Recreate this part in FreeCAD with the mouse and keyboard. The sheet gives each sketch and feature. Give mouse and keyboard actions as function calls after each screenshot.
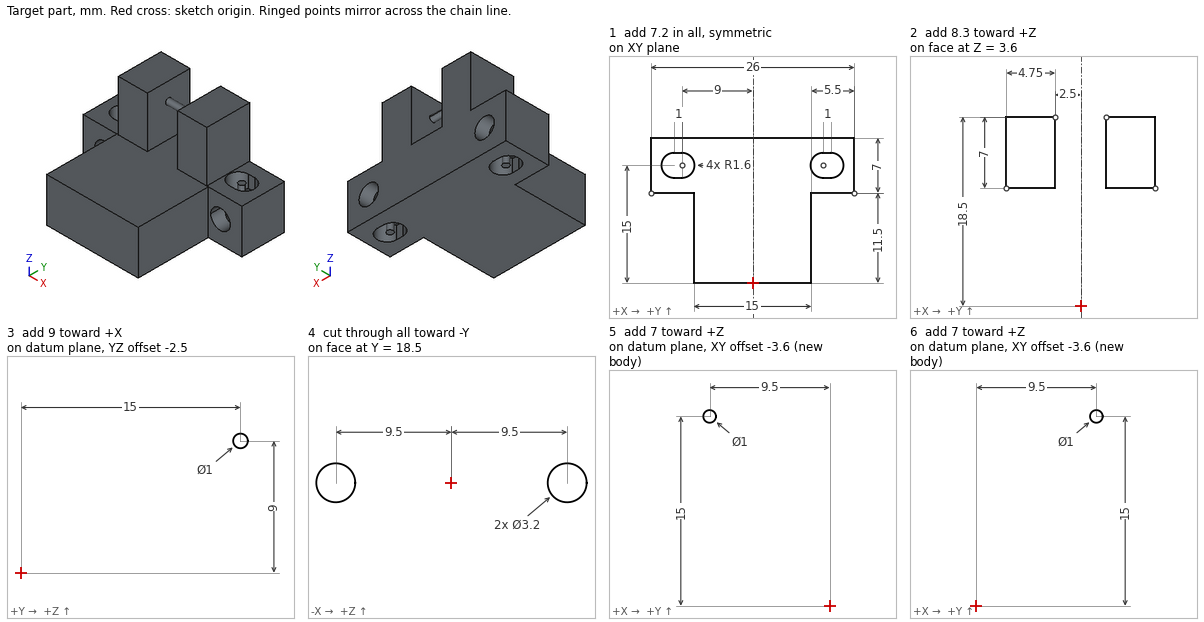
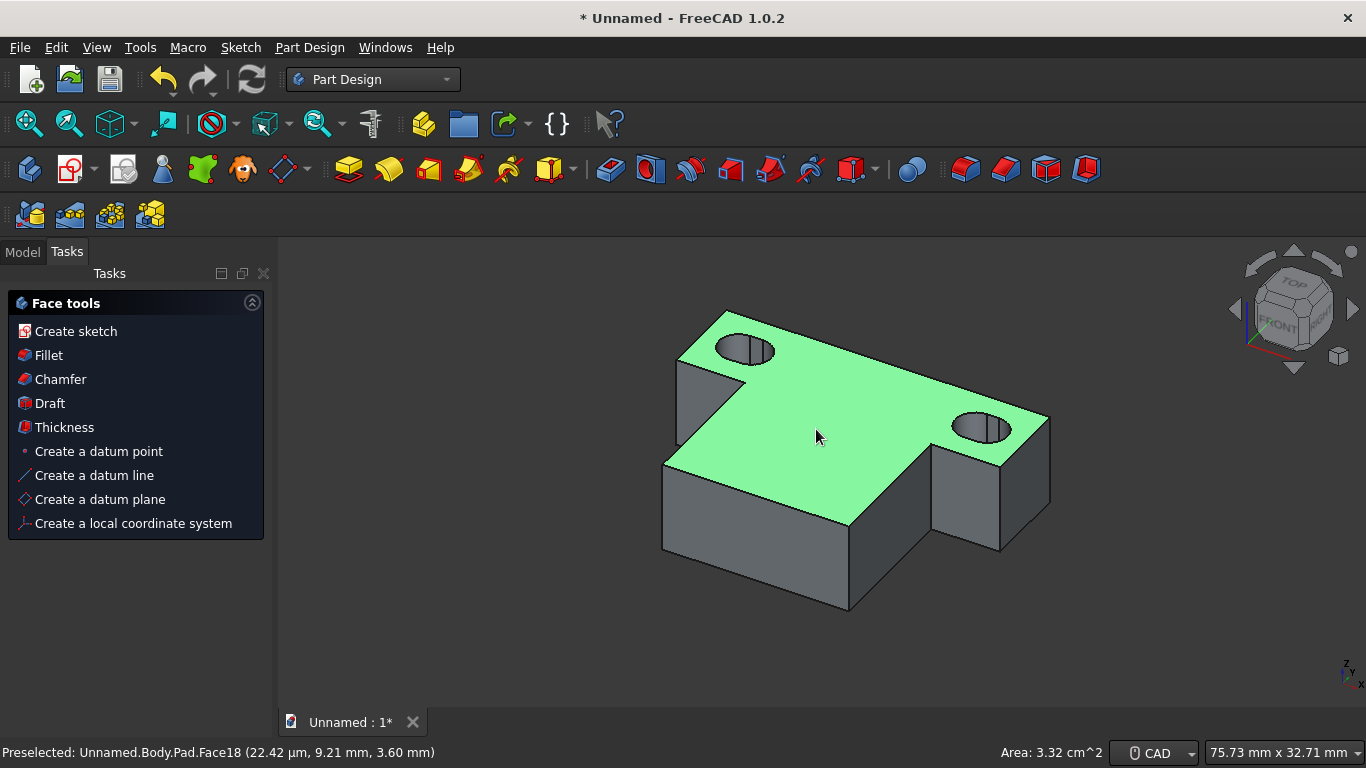
click(70, 170)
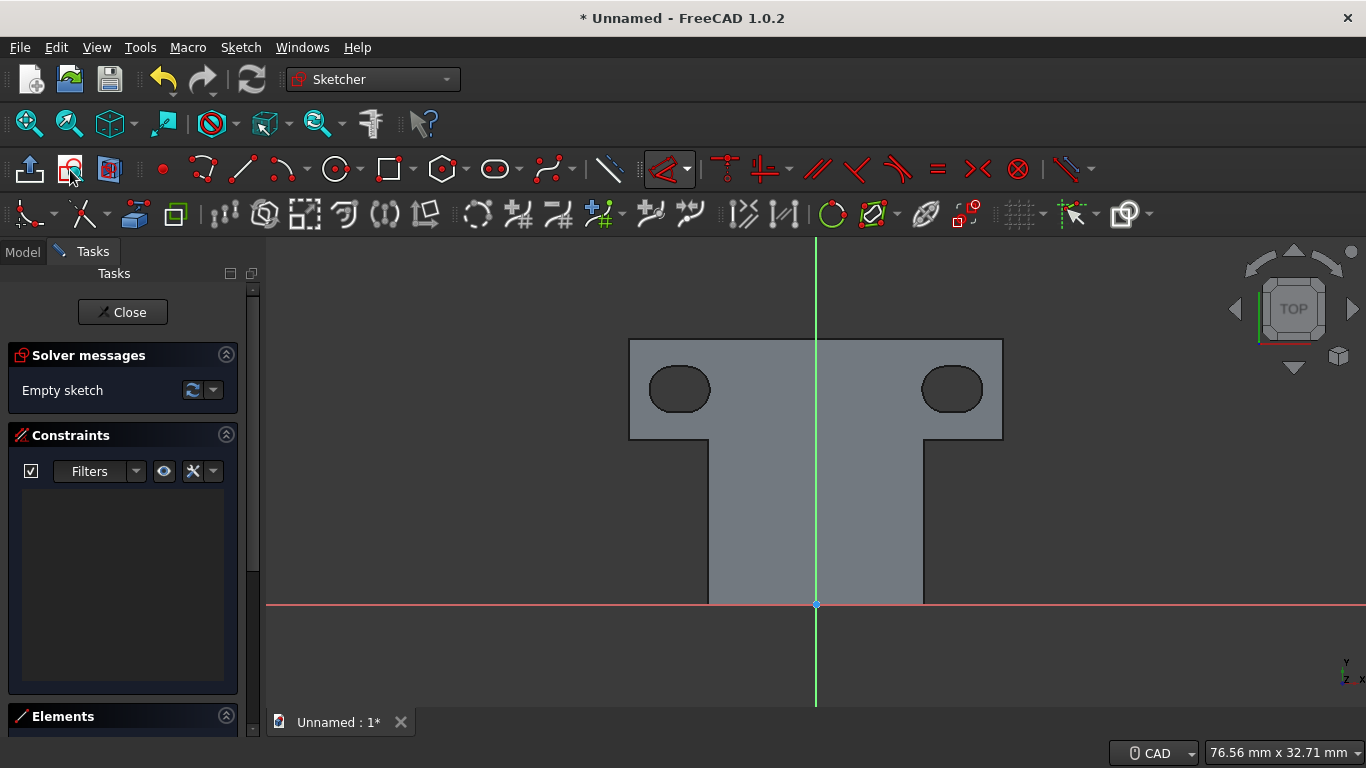
click(390, 170)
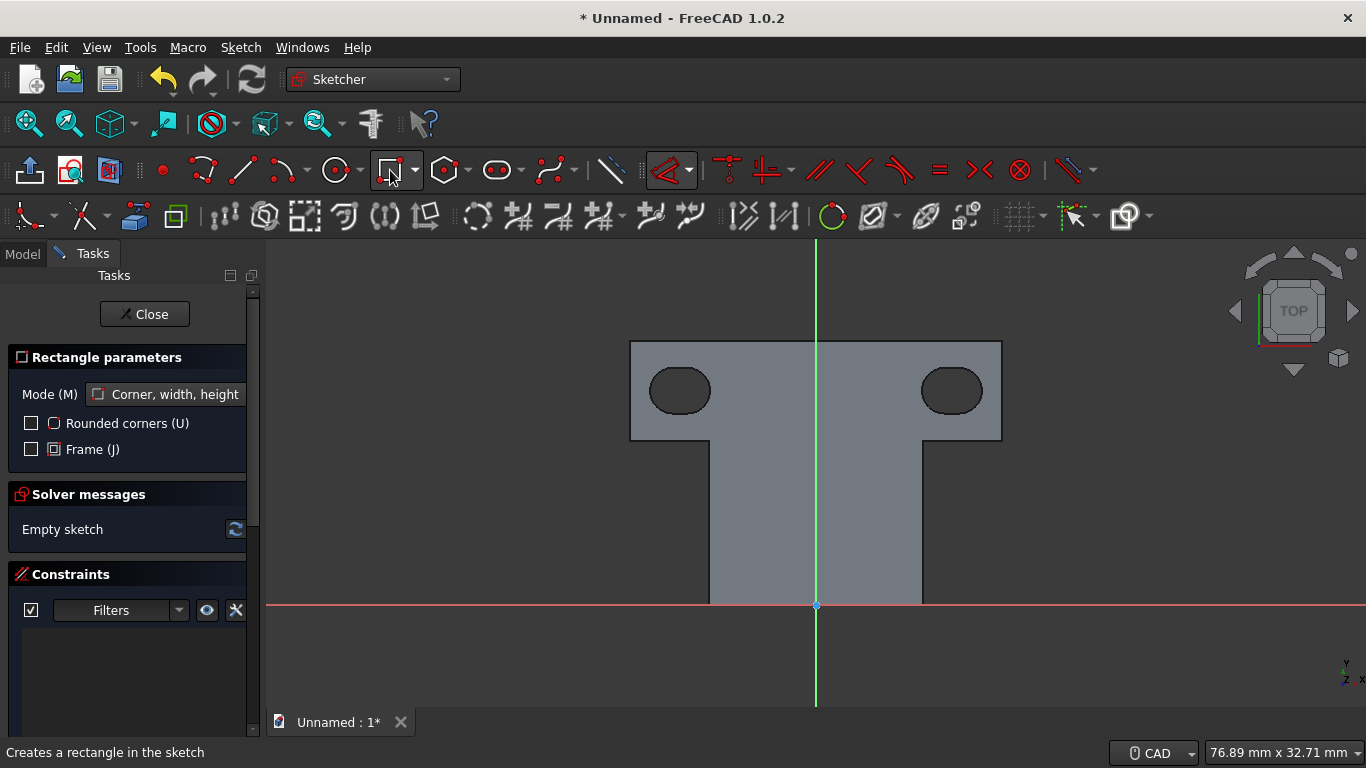
click(712, 341)
click(780, 441)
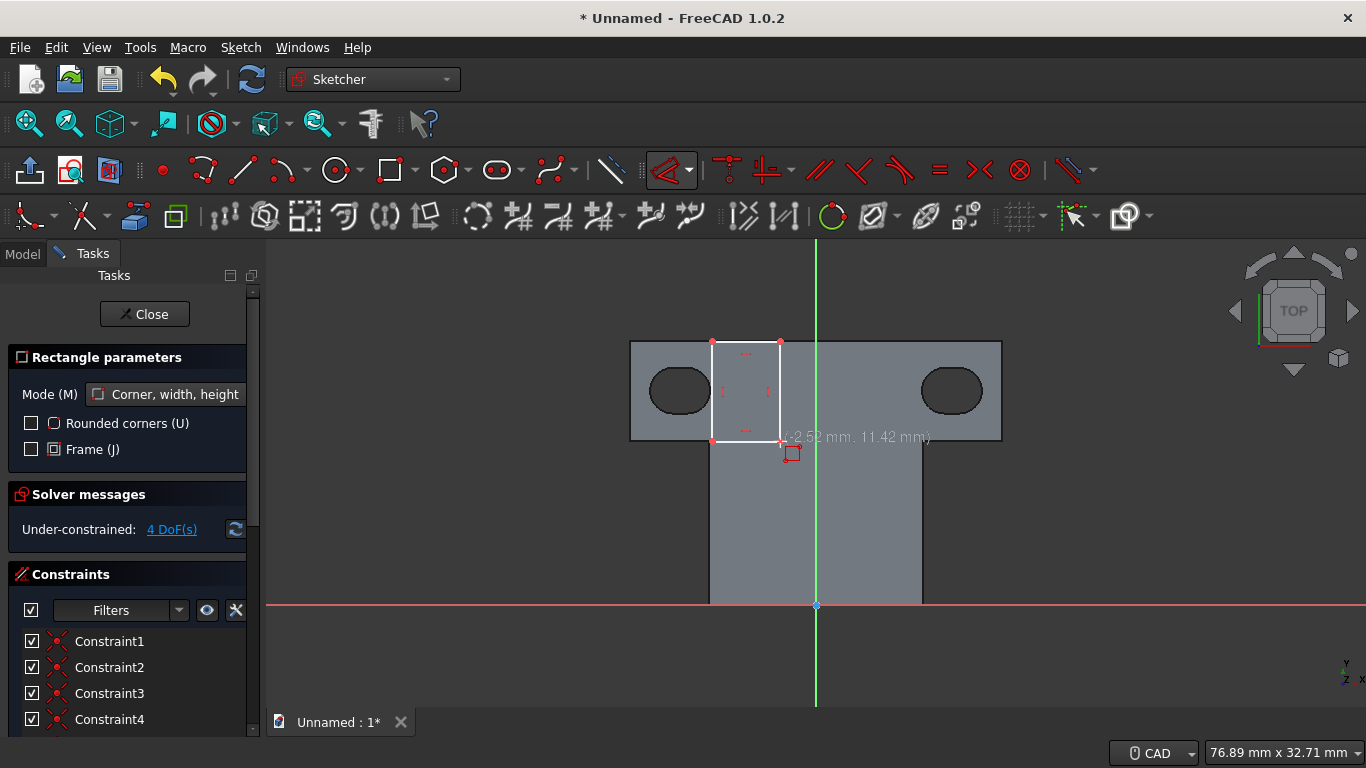
click(852, 341)
click(920, 441)
key(Escape)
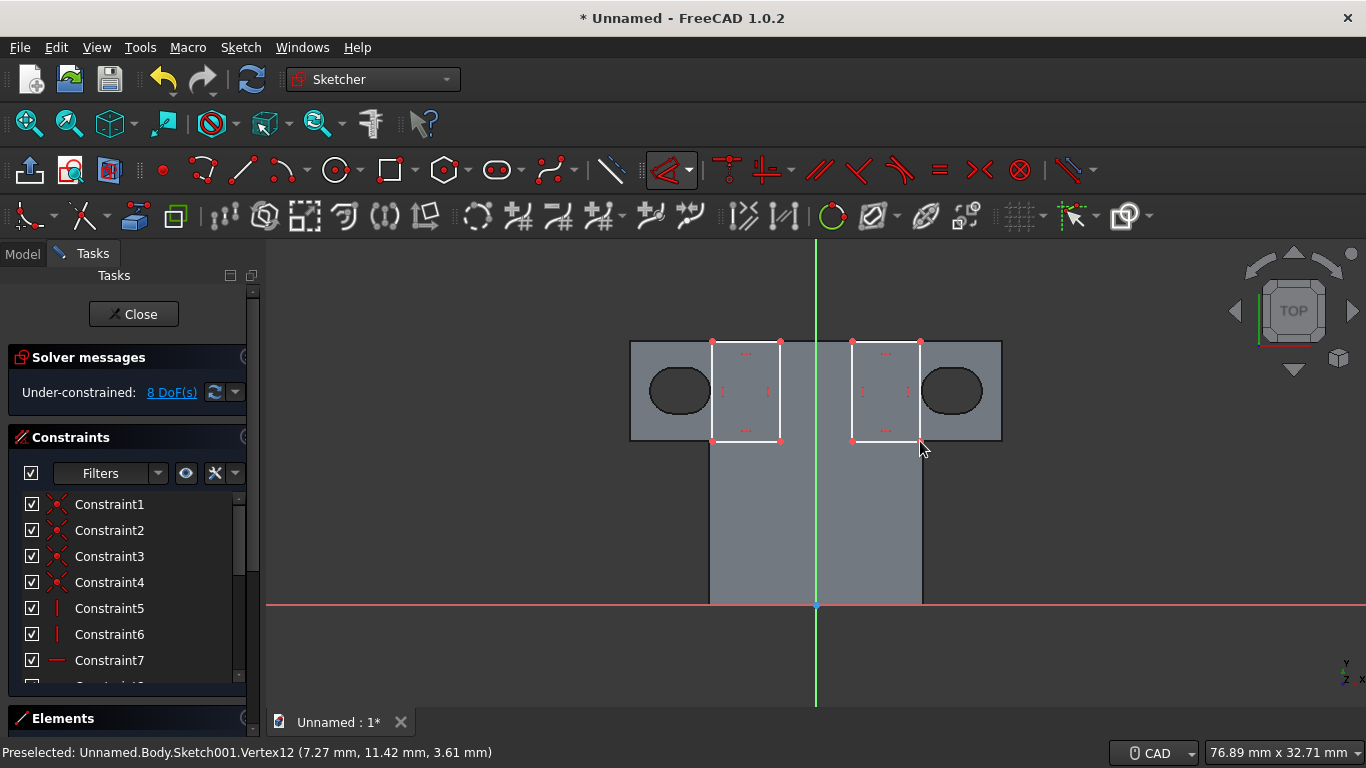
click(780, 342)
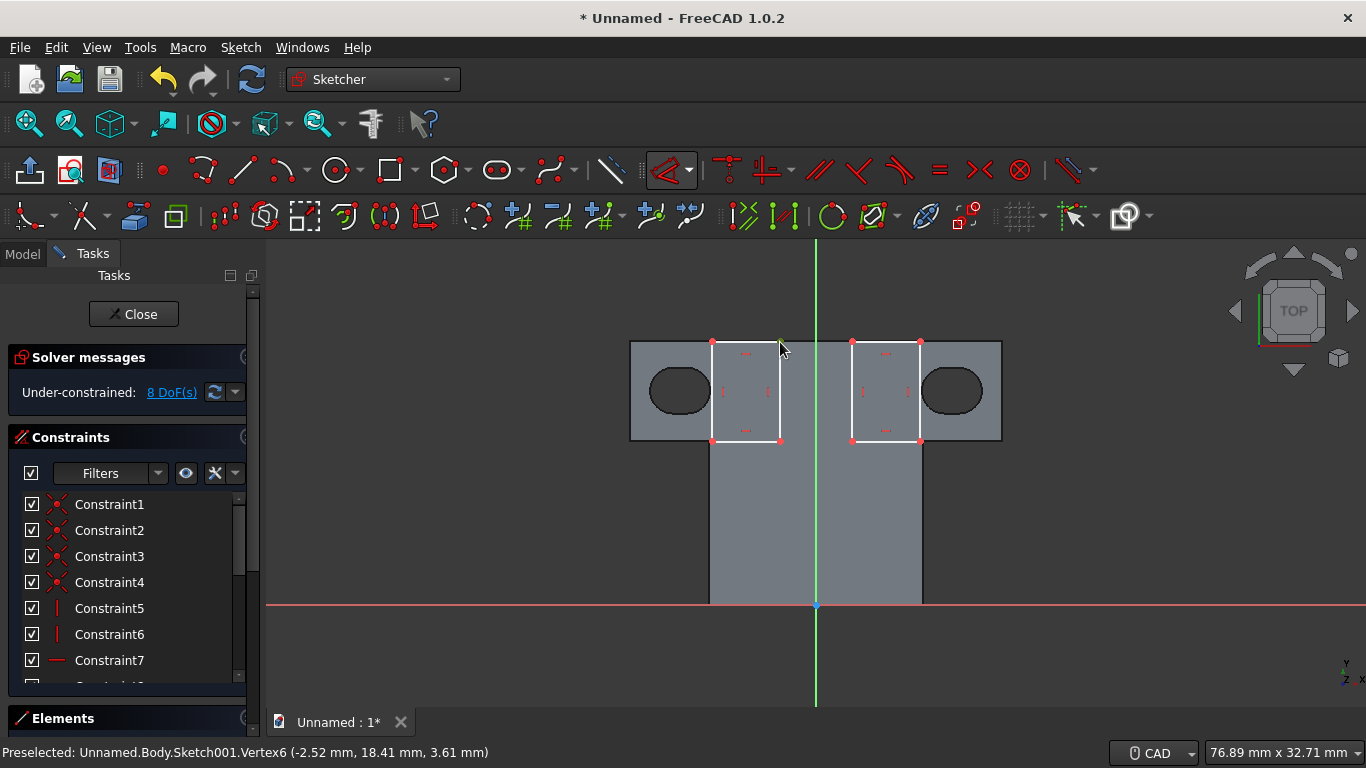
click(852, 342)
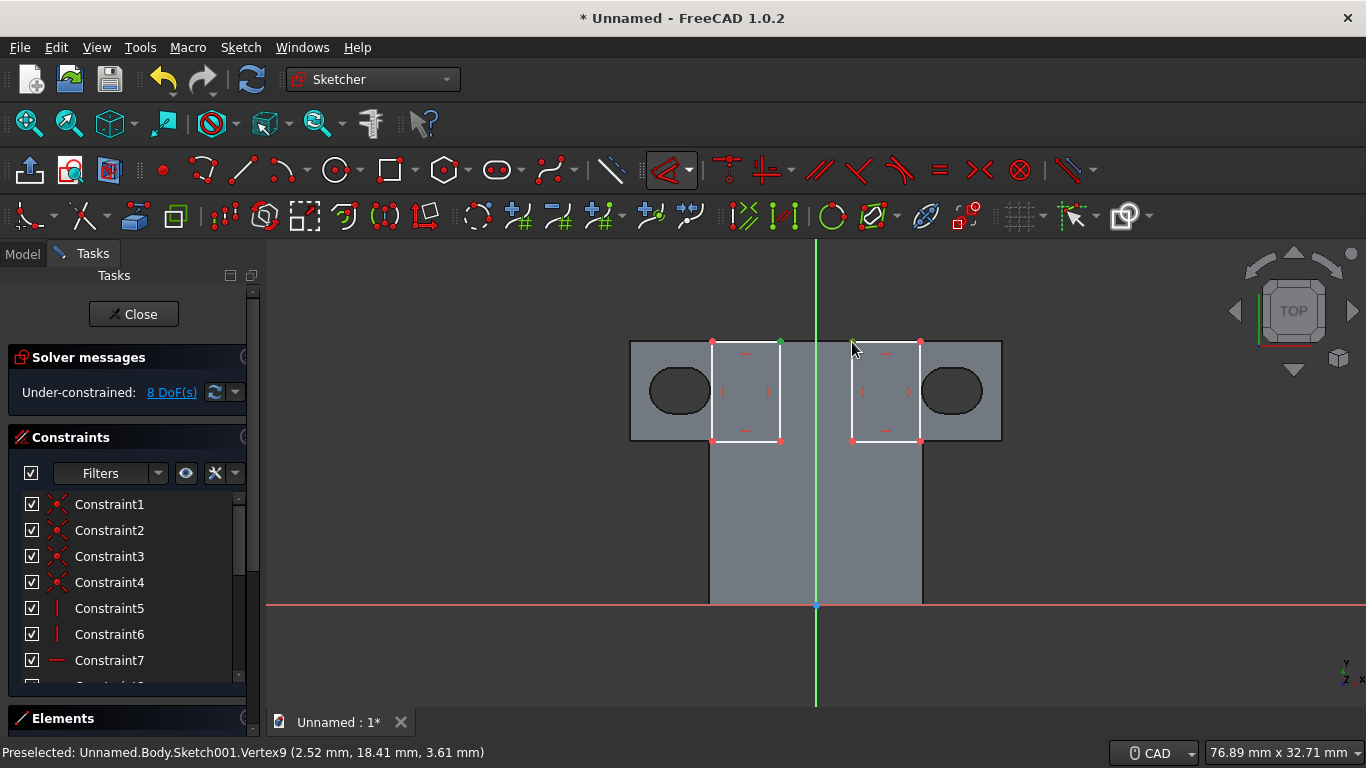
click(816, 650)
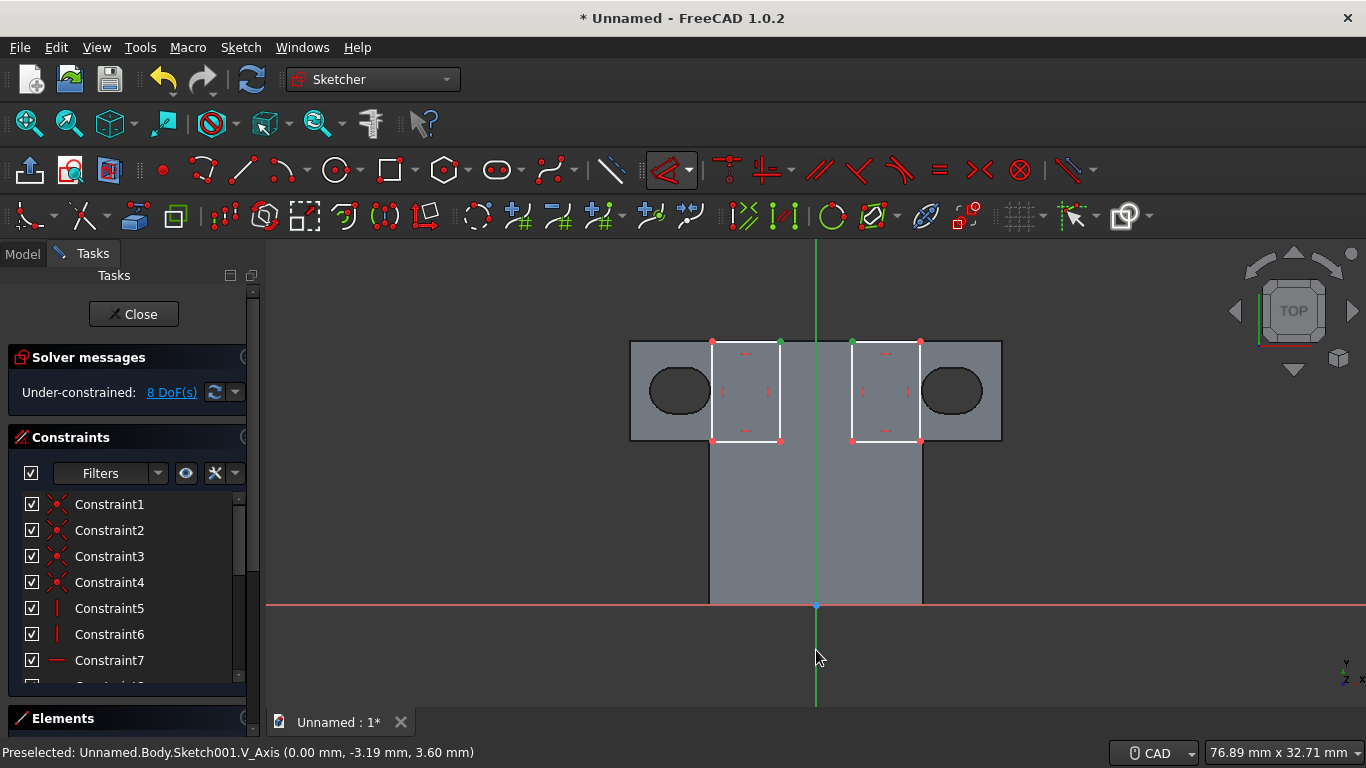
key(s)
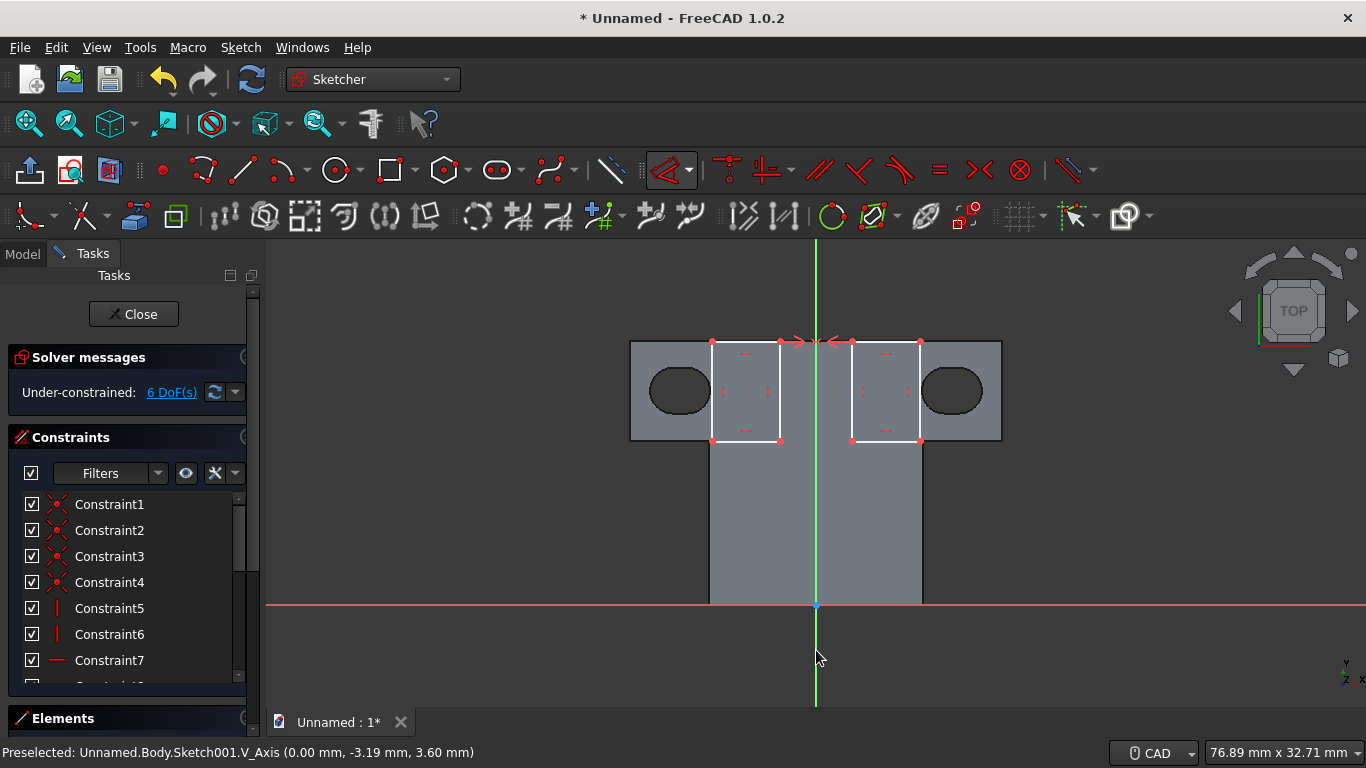
click(712, 442)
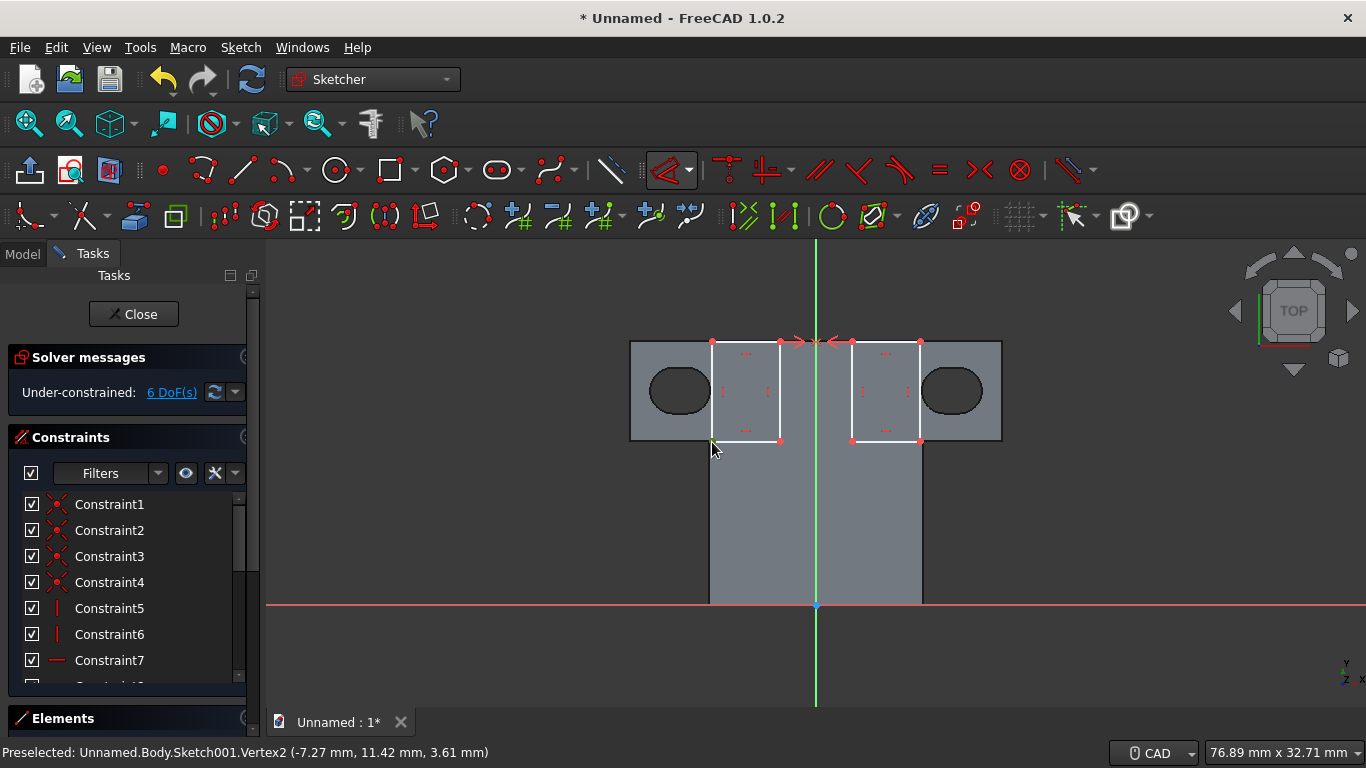
click(920, 442)